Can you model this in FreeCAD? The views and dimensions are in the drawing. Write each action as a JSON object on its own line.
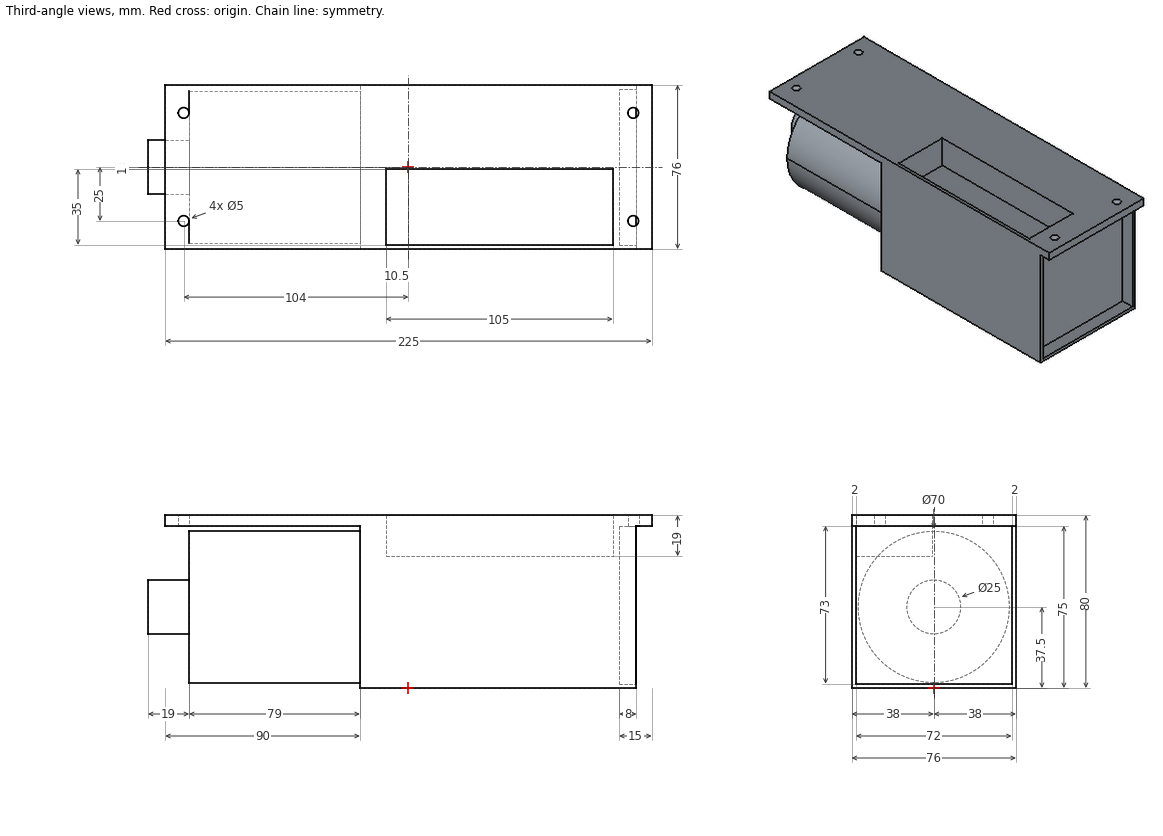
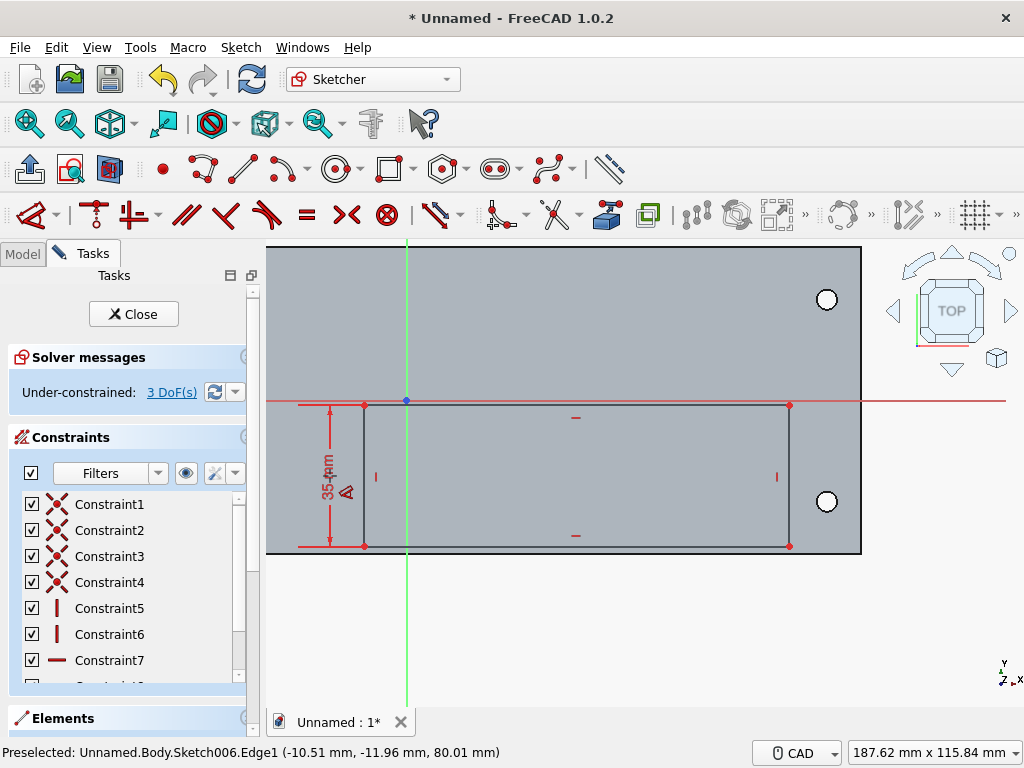
{"action": "scroll", "coordinate": [364, 405], "scroll_direction": "up", "scroll_amount": 12}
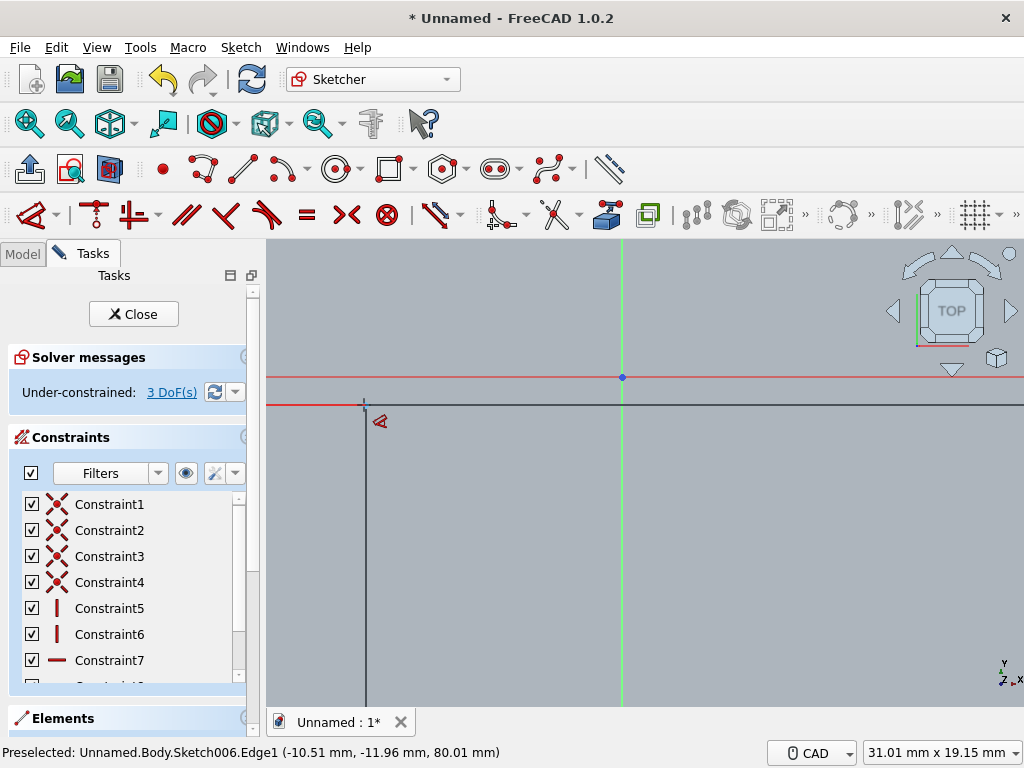
{"action": "left_click", "coordinate": [367, 405]}
{"action": "left_click", "coordinate": [333, 379]}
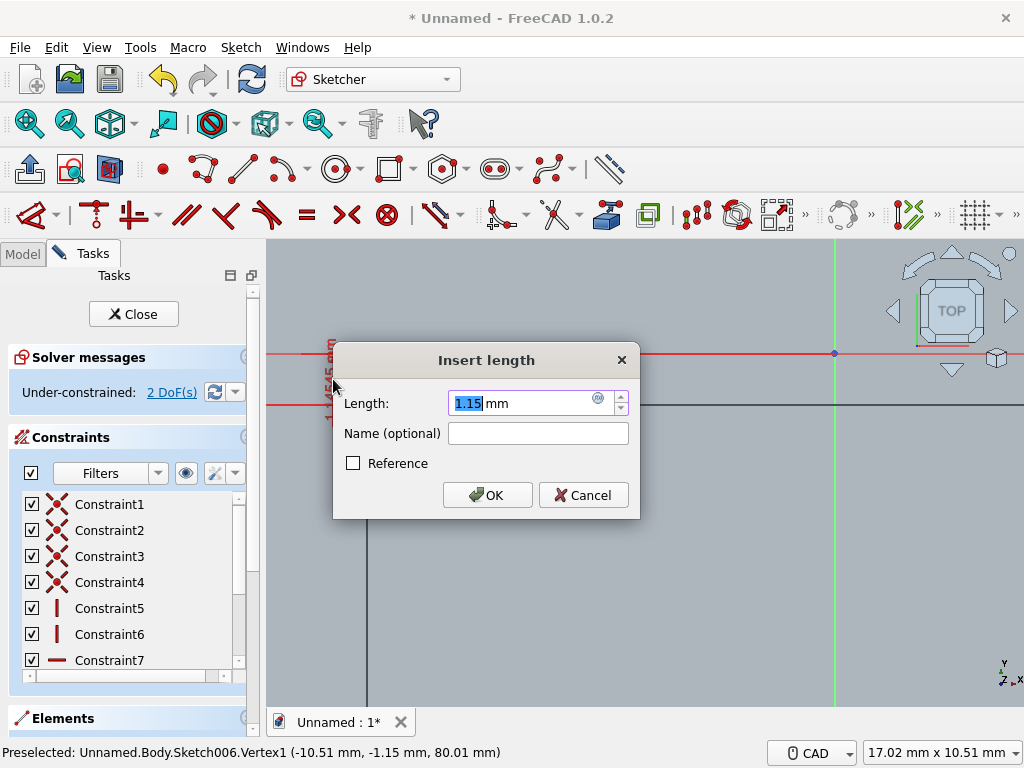
{"action": "type", "text": "1"}
{"action": "key", "text": "Return"}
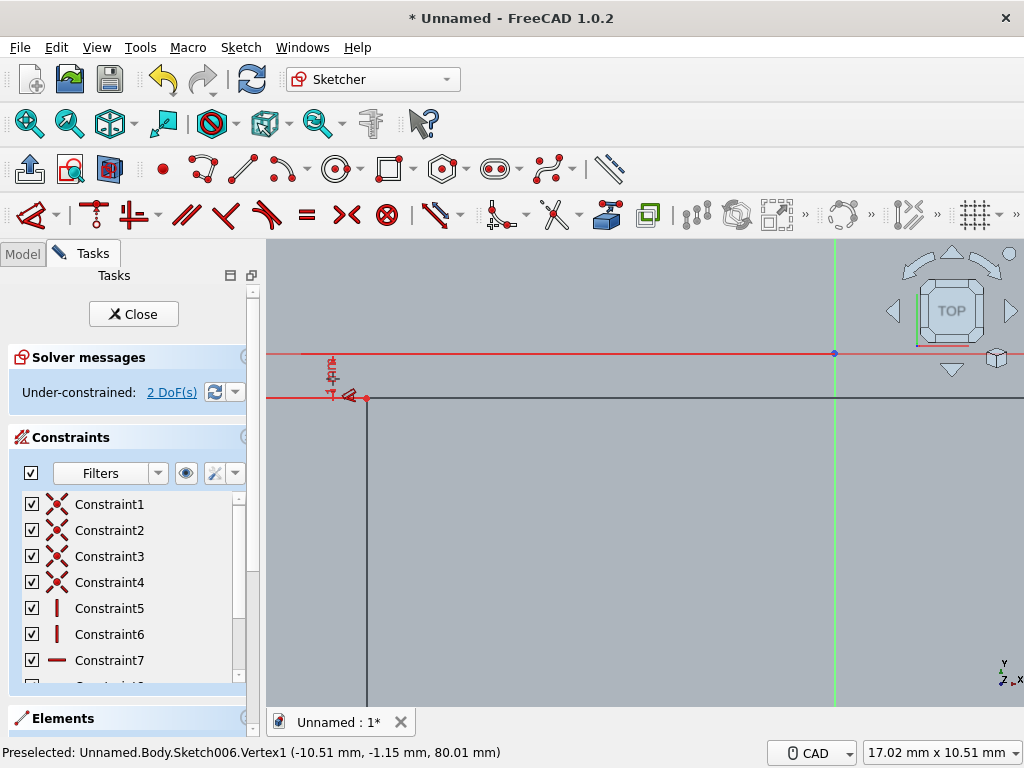
{"action": "scroll", "coordinate": [364, 405], "scroll_direction": "down", "scroll_amount": 12}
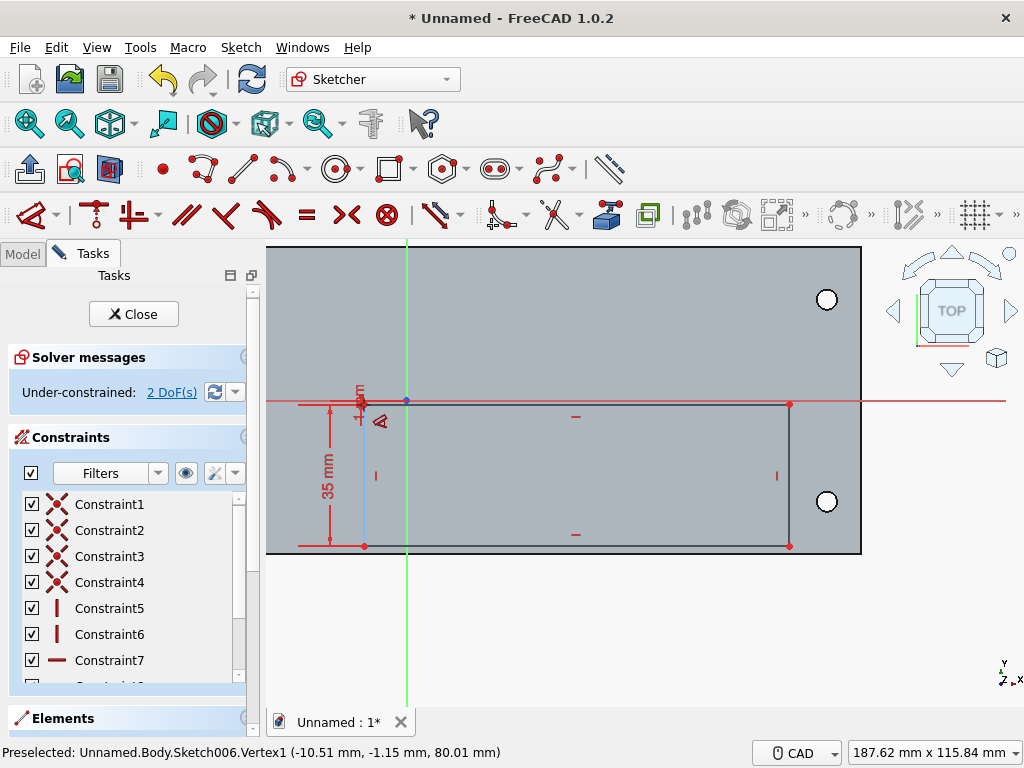
{"action": "left_click", "coordinate": [492, 546]}
{"action": "left_click", "coordinate": [577, 580]}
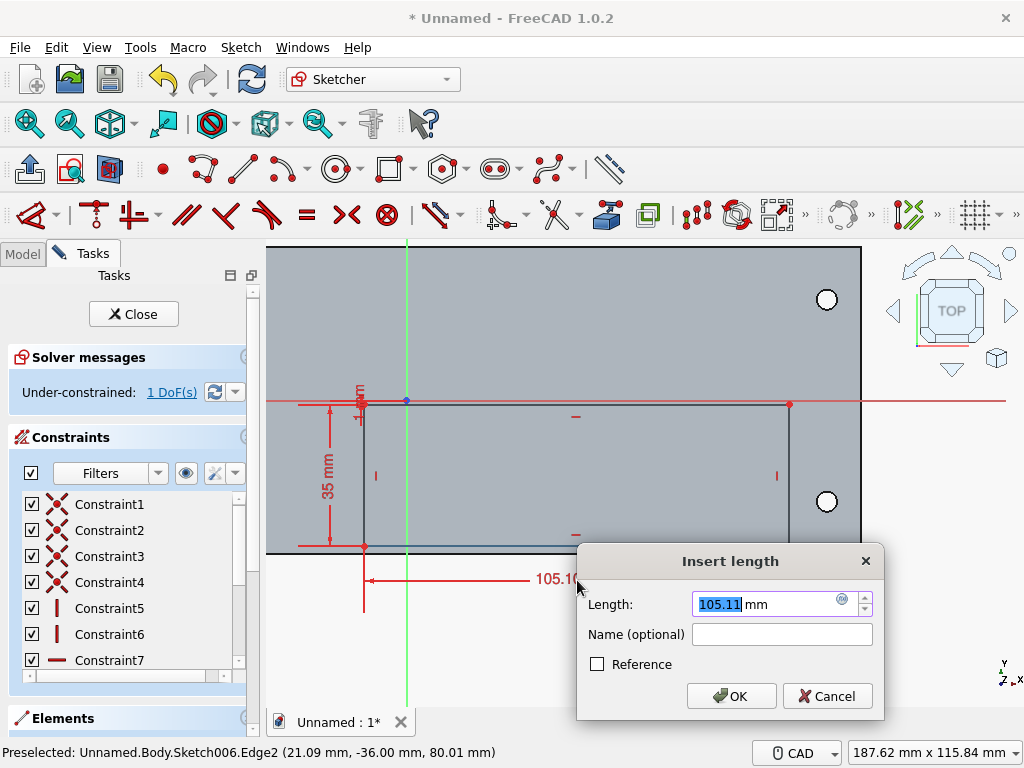
{"action": "type", "text": "105"}
{"action": "key", "text": "Return"}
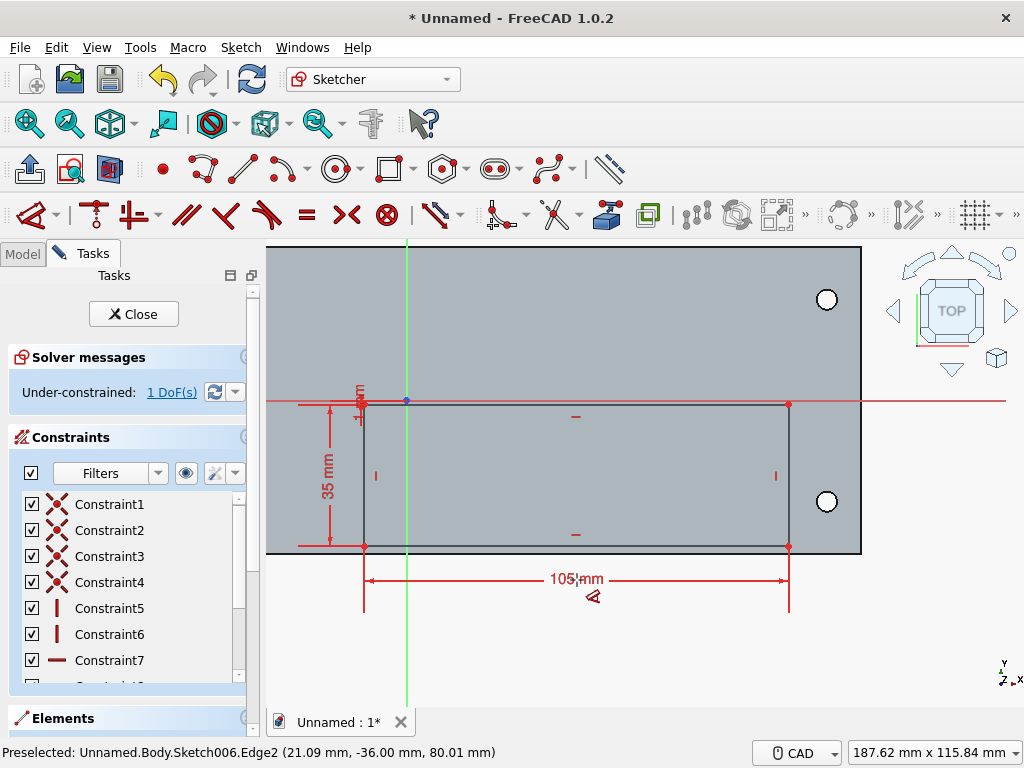
{"action": "left_click", "coordinate": [364, 405]}
{"action": "left_click", "coordinate": [386, 367]}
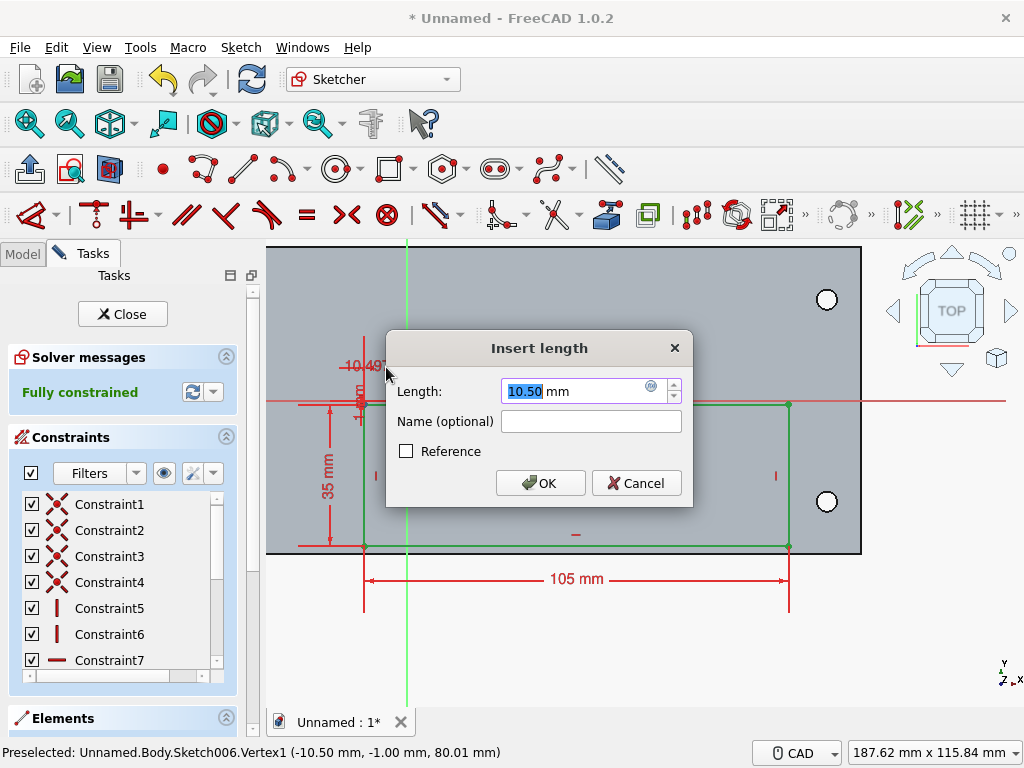
{"action": "type", "text": "10.5"}
{"action": "key", "text": "Return"}
{"action": "key", "text": "Escape"}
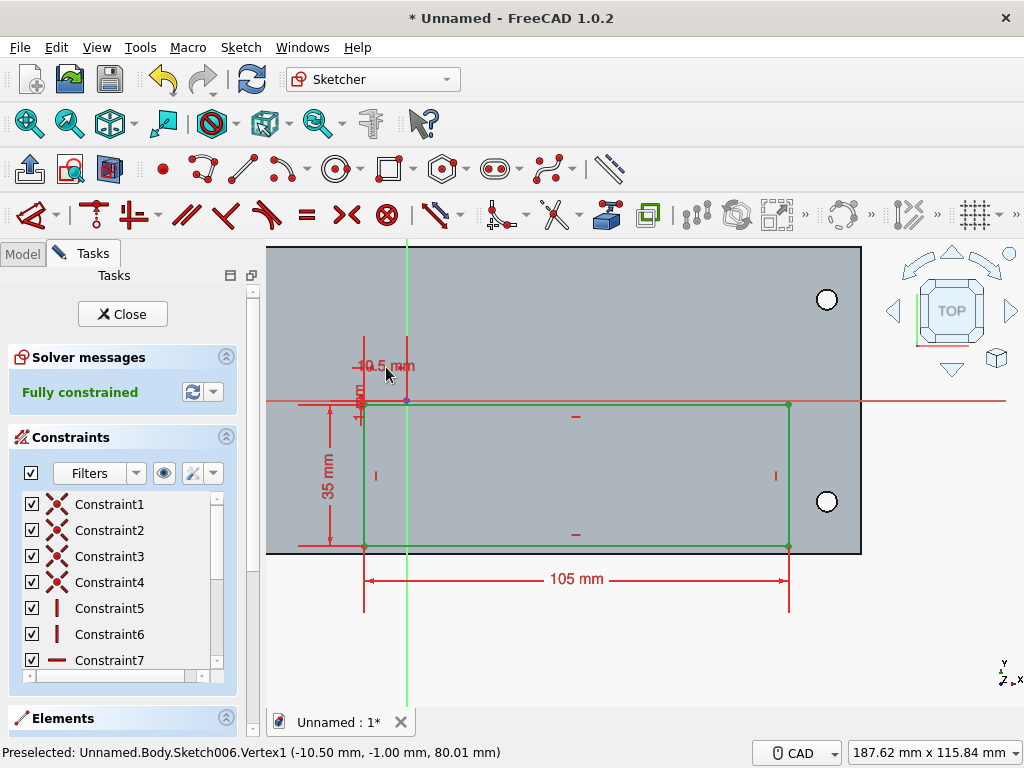
{"action": "left_click", "coordinate": [123, 314]}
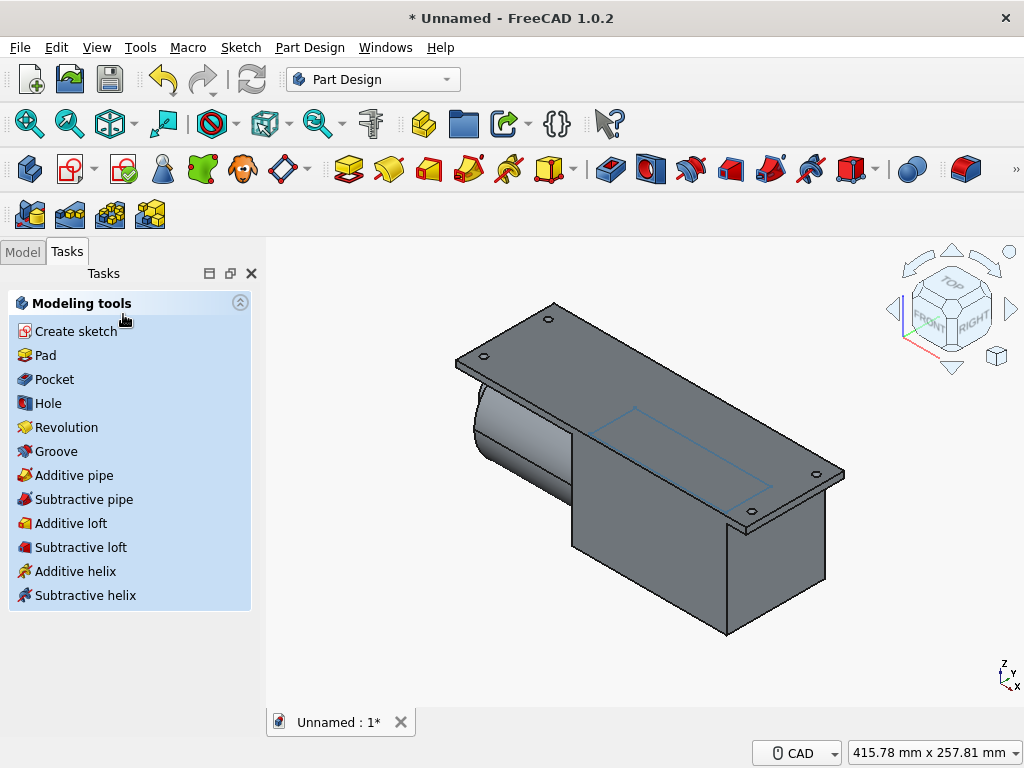
{"action": "left_click", "coordinate": [612, 170]}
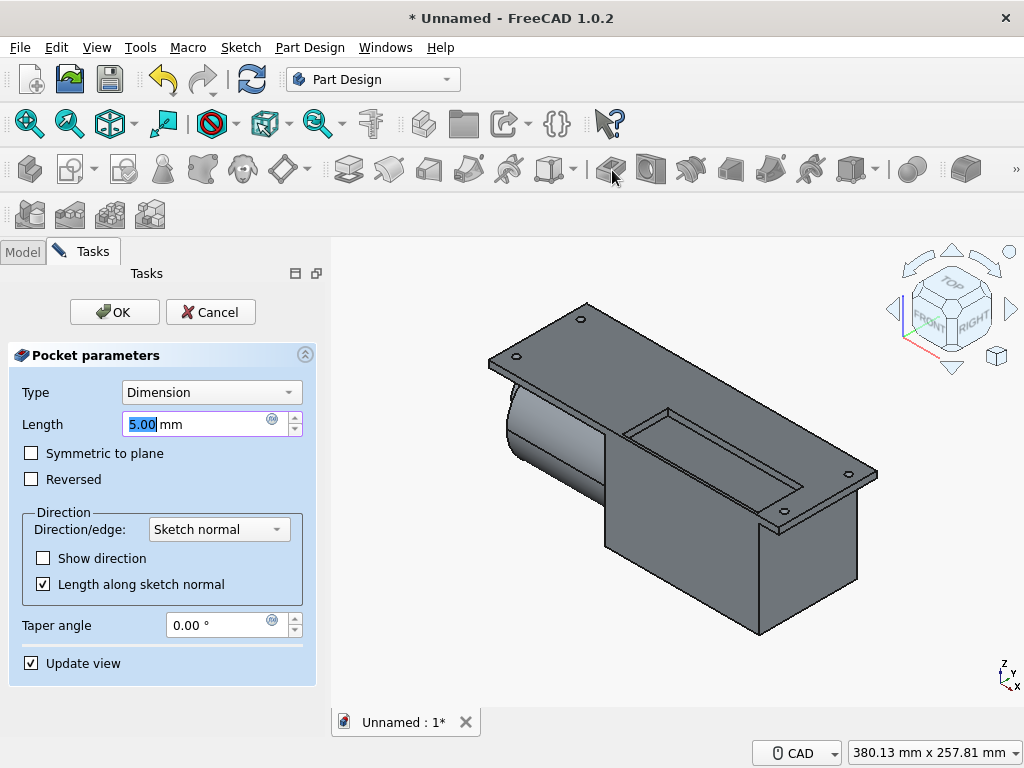
{"action": "type", "text": "19"}
{"action": "key", "text": "Tab"}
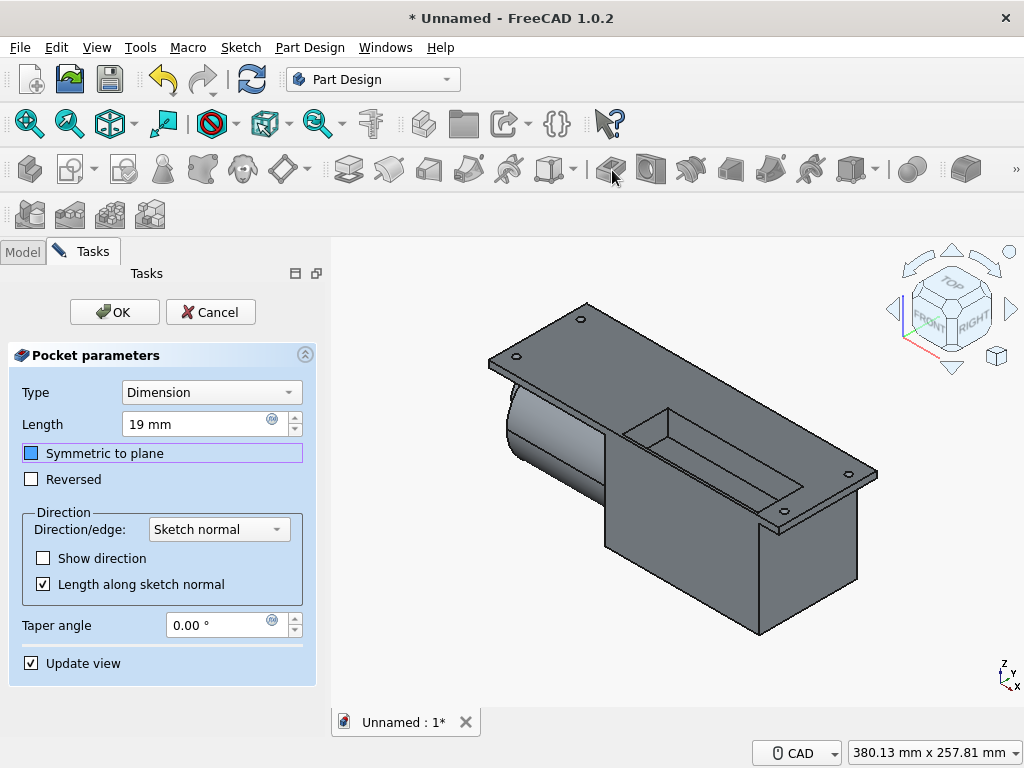
{"action": "left_click", "coordinate": [115, 312]}